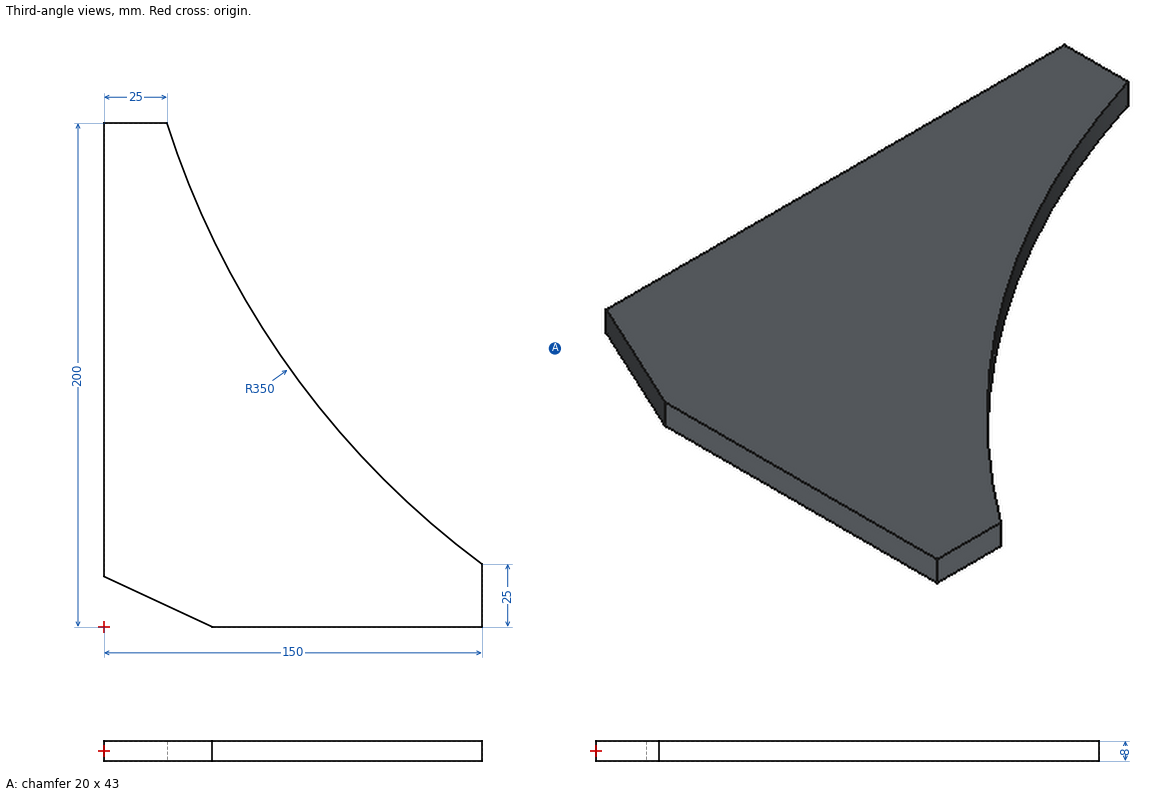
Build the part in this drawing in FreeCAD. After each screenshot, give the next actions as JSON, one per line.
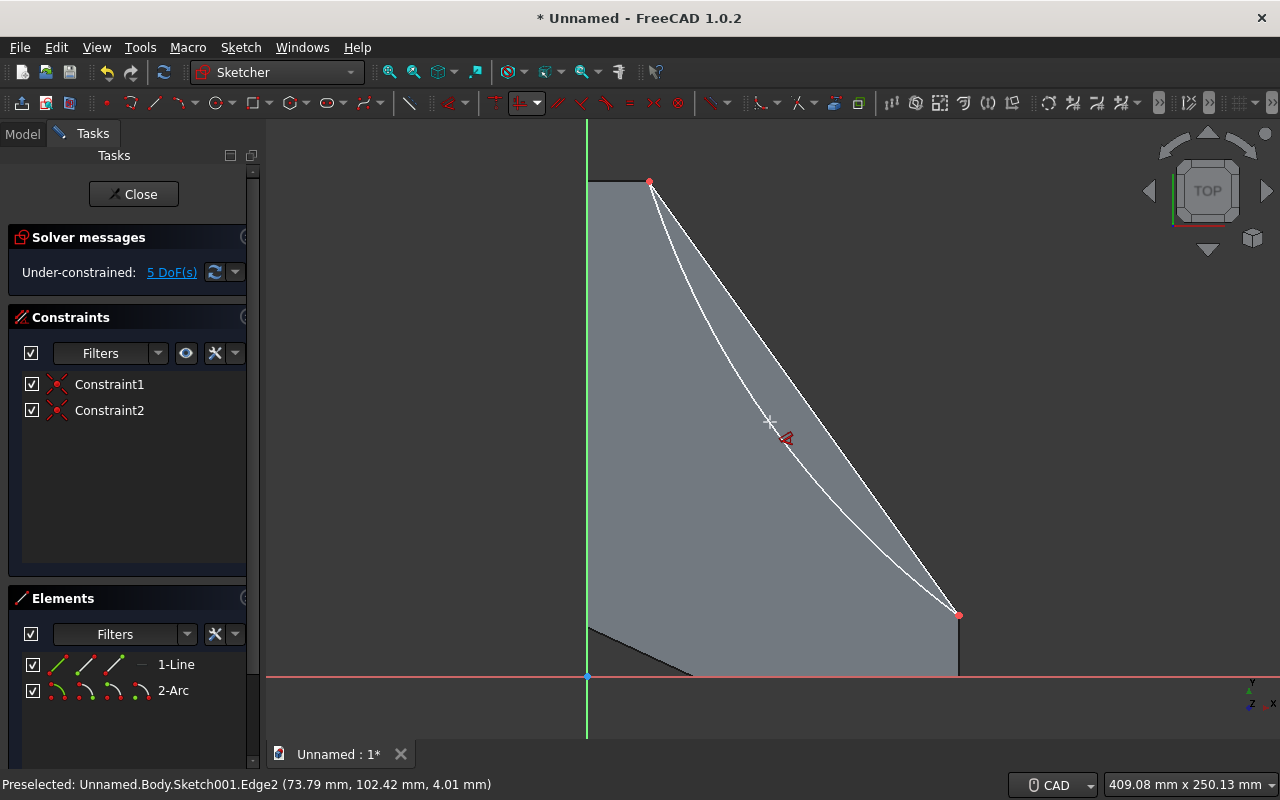
{"action": "left_click", "coordinate": [713, 331]}
{"action": "left_click", "coordinate": [685, 346]}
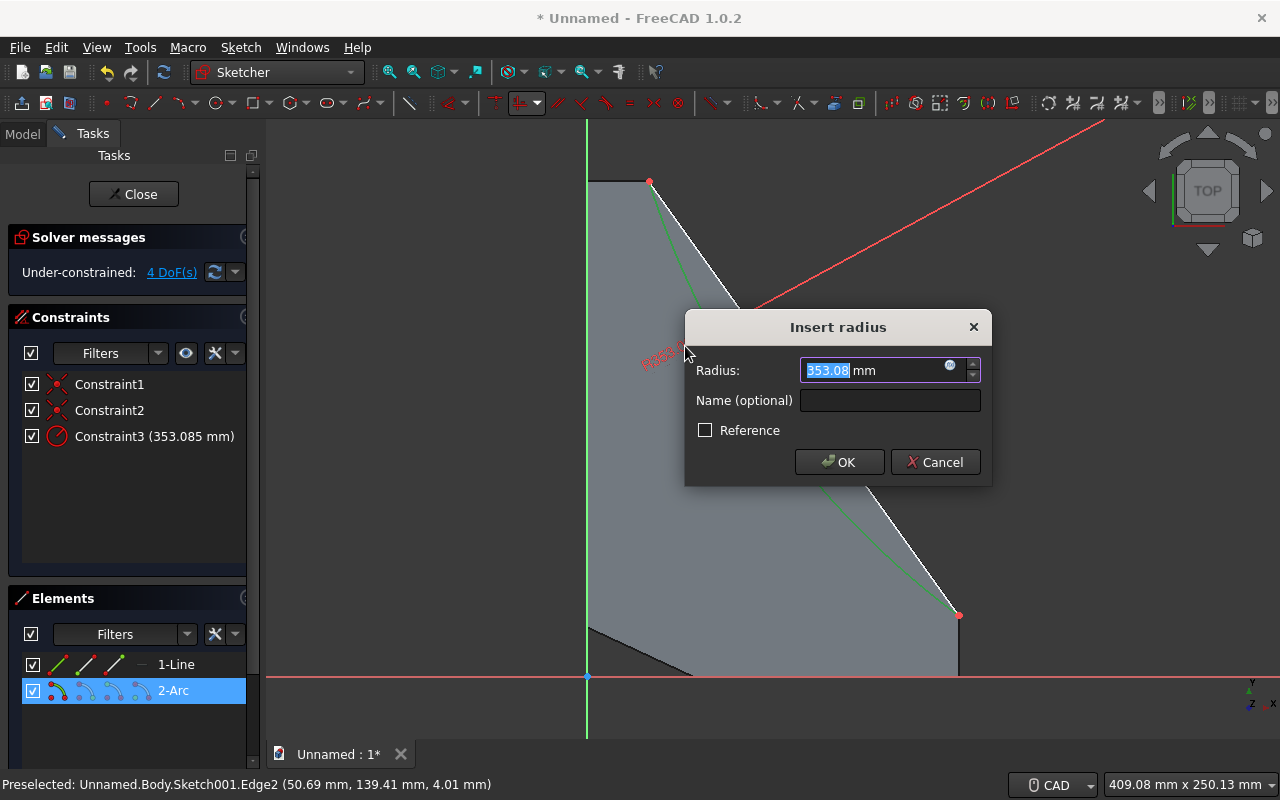
{"action": "type", "text": "350"}
{"action": "key", "text": "Return"}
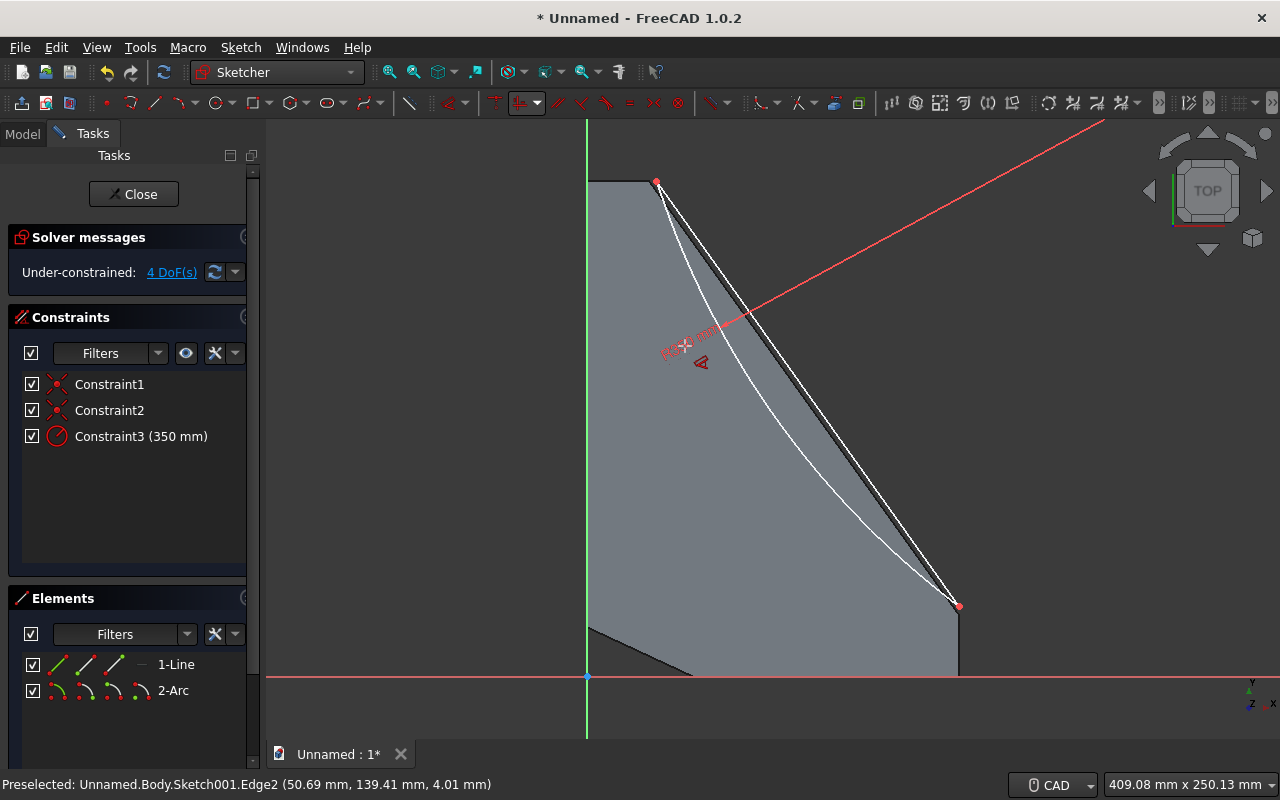
{"action": "left_click", "coordinate": [959, 607]}
{"action": "left_click", "coordinate": [993, 642]}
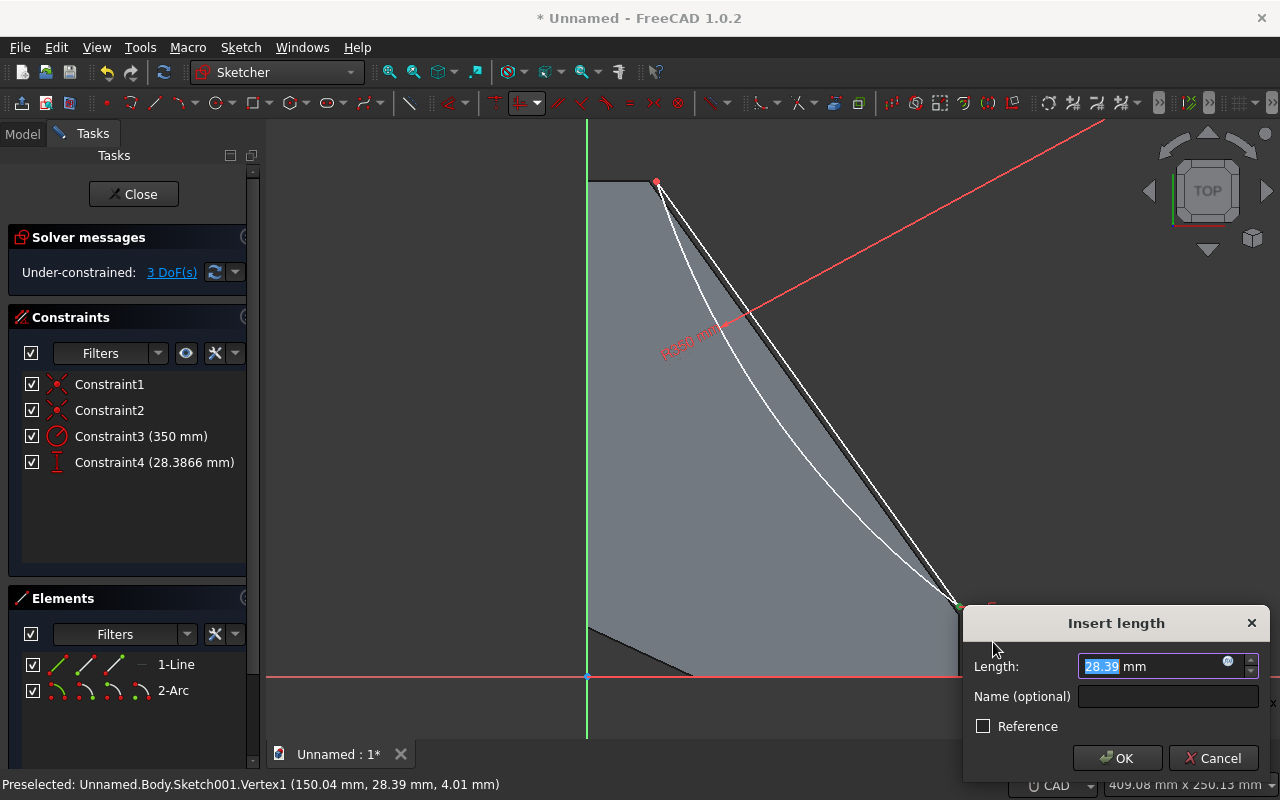
{"action": "type", "text": "25"}
{"action": "key", "text": "Return"}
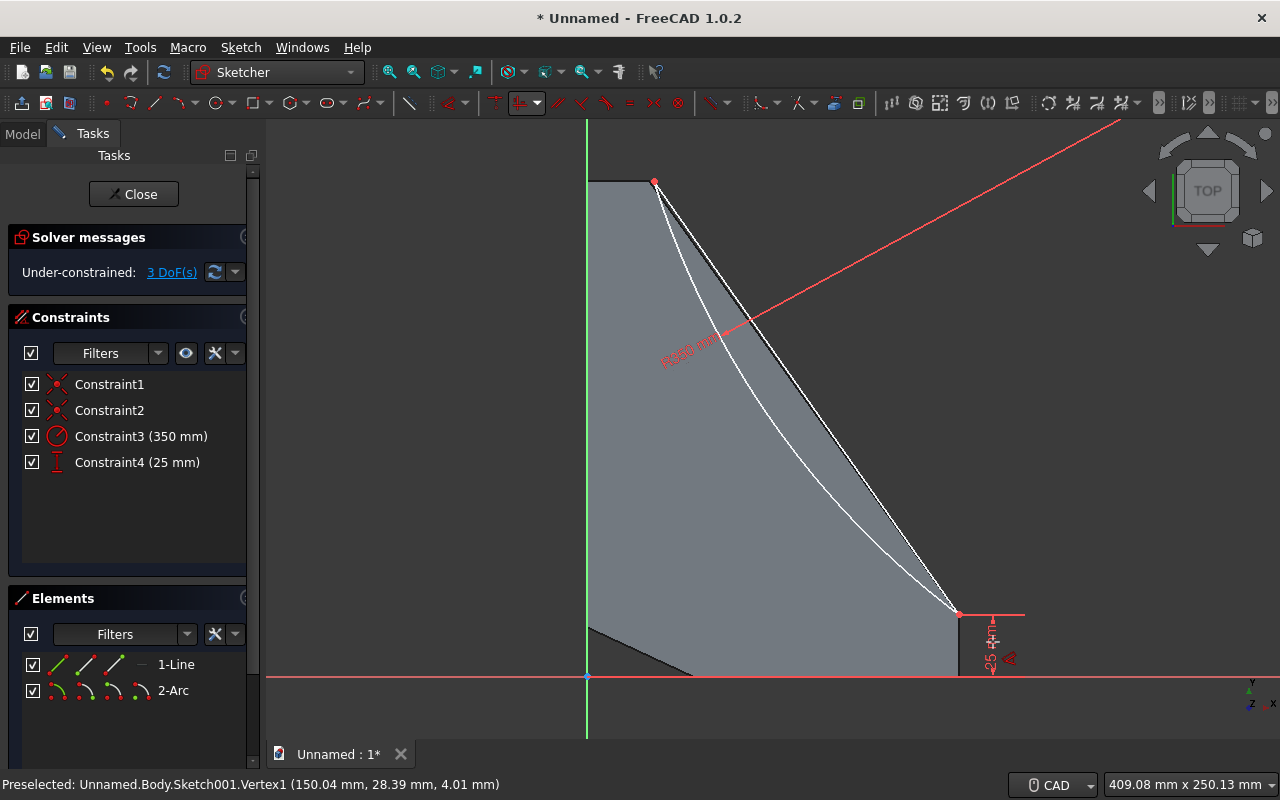
{"action": "left_click", "coordinate": [654, 182]}
{"action": "left_click", "coordinate": [621, 711]}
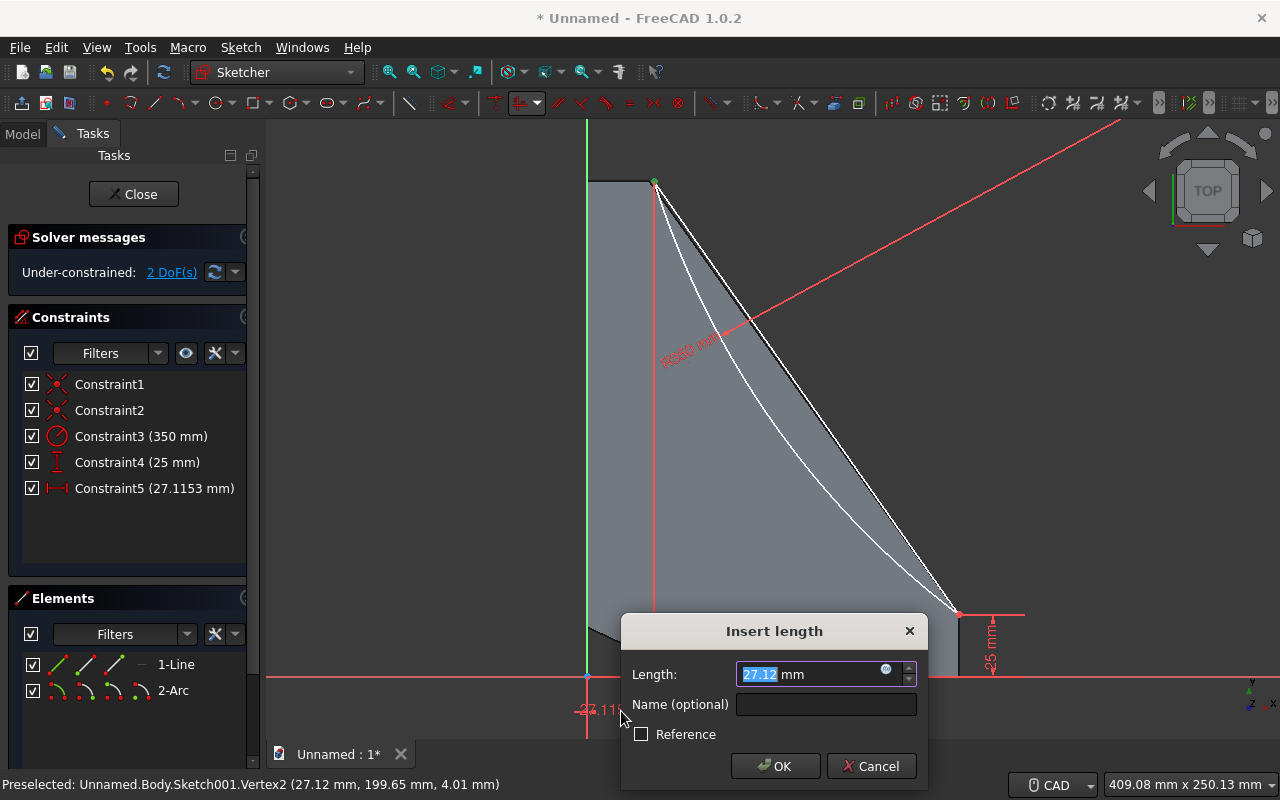
{"action": "type", "text": "25"}
{"action": "key", "text": "Return"}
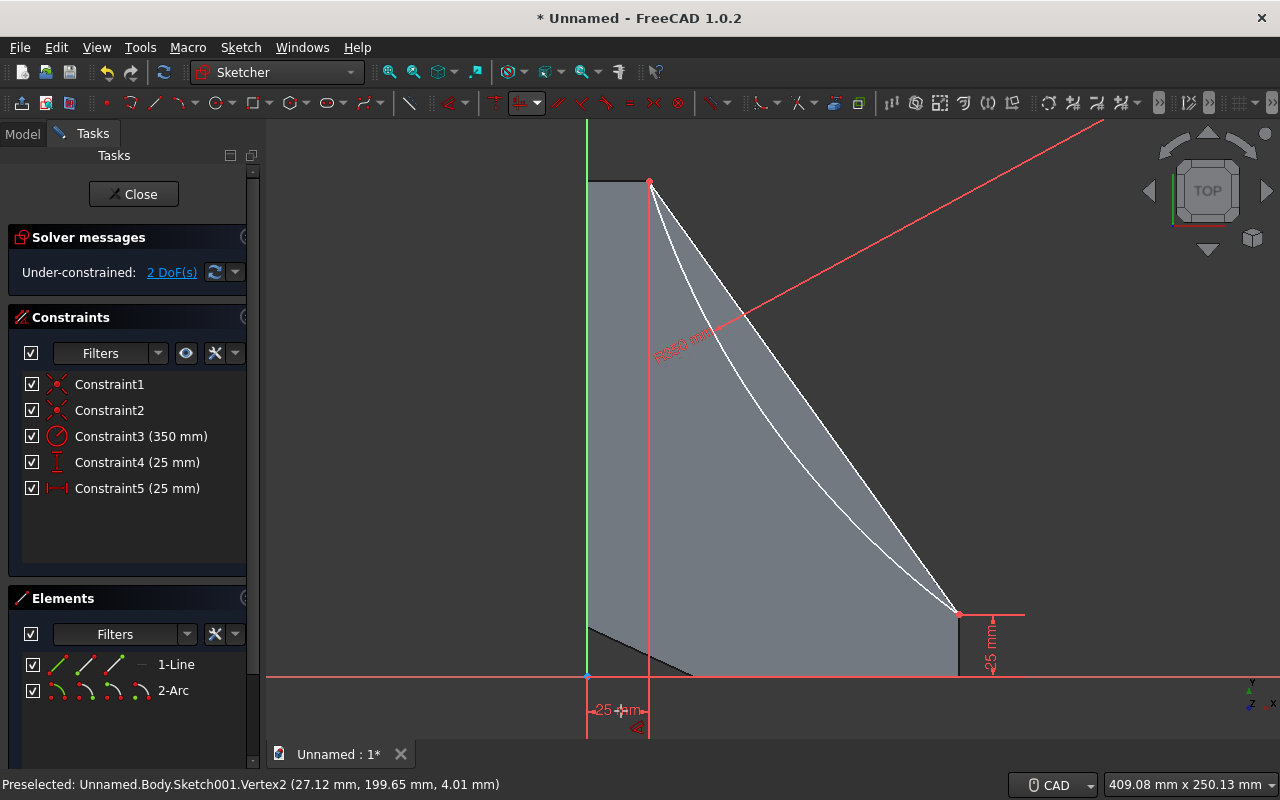
{"action": "left_click", "coordinate": [959, 615]}
{"action": "left_click", "coordinate": [773, 711]}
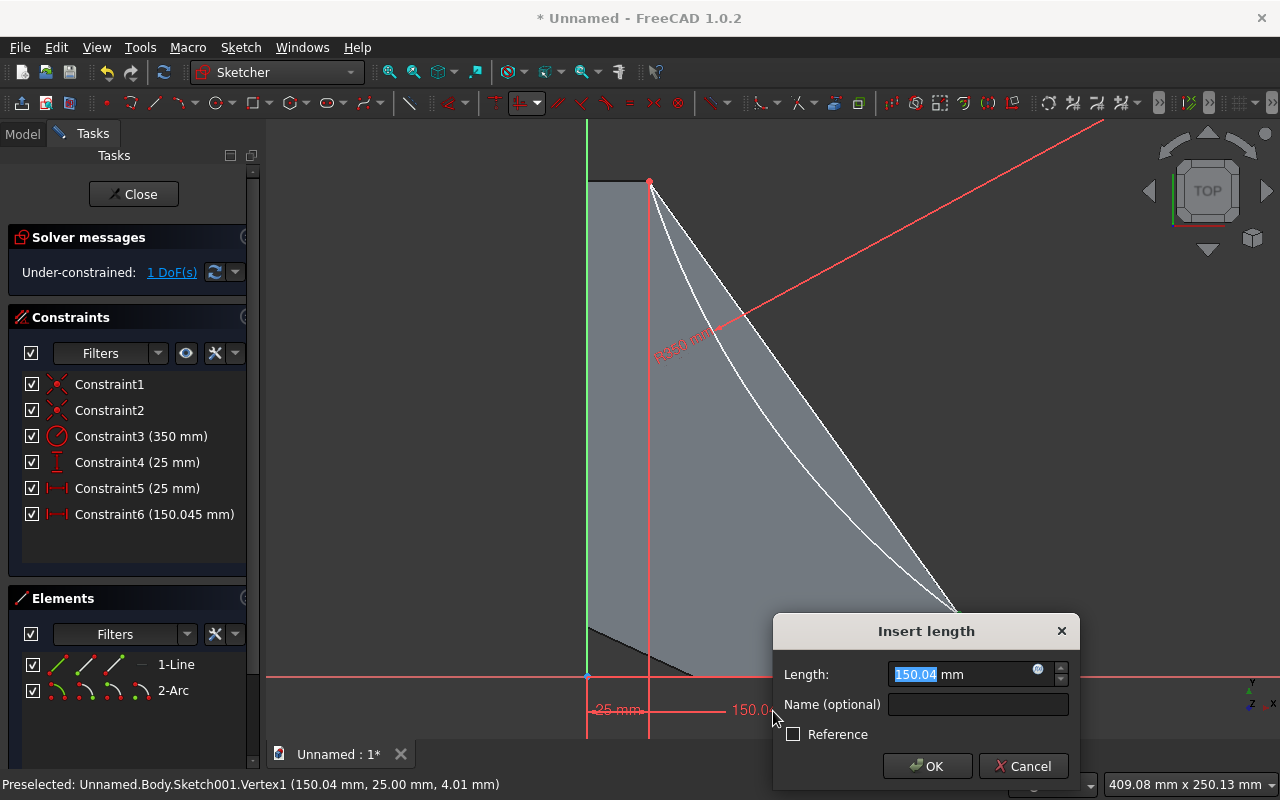
{"action": "type", "text": "150"}
{"action": "key", "text": "Return"}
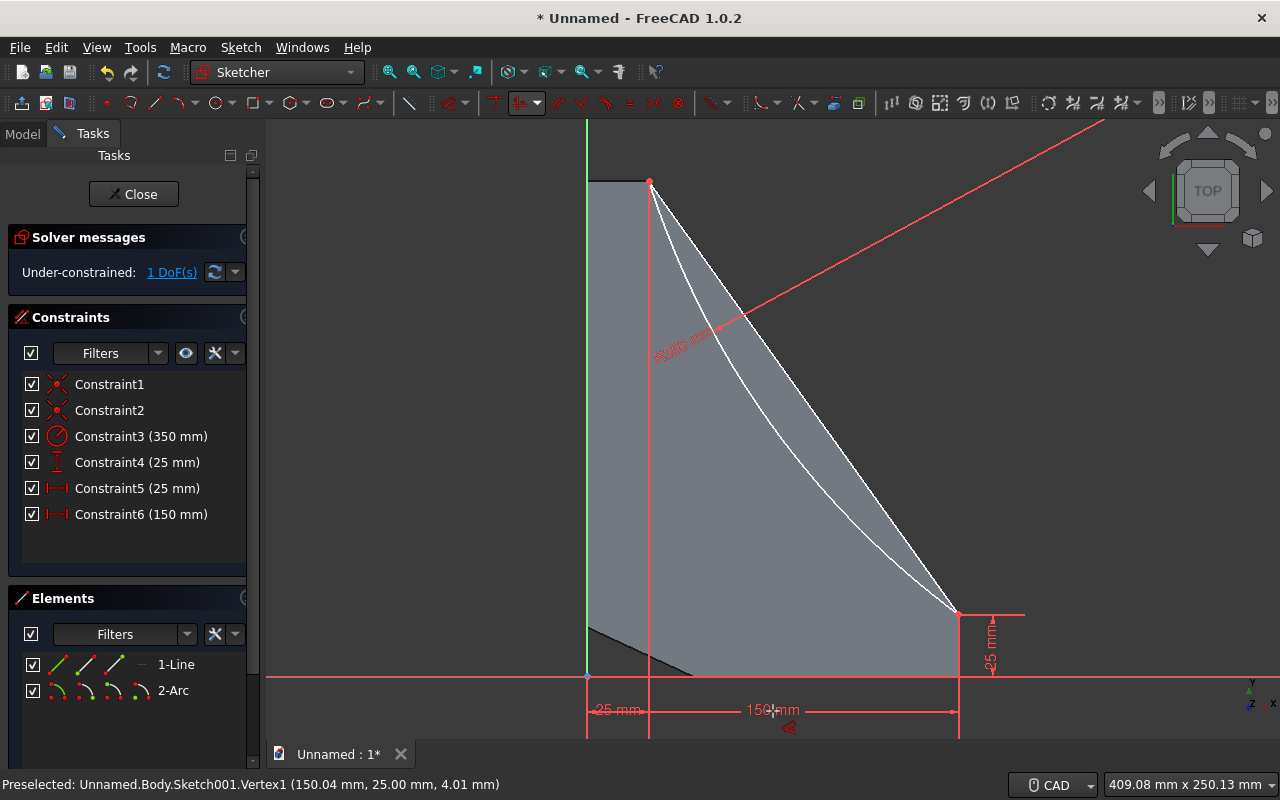
{"action": "left_click", "coordinate": [649, 182]}
{"action": "left_click", "coordinate": [553, 429]}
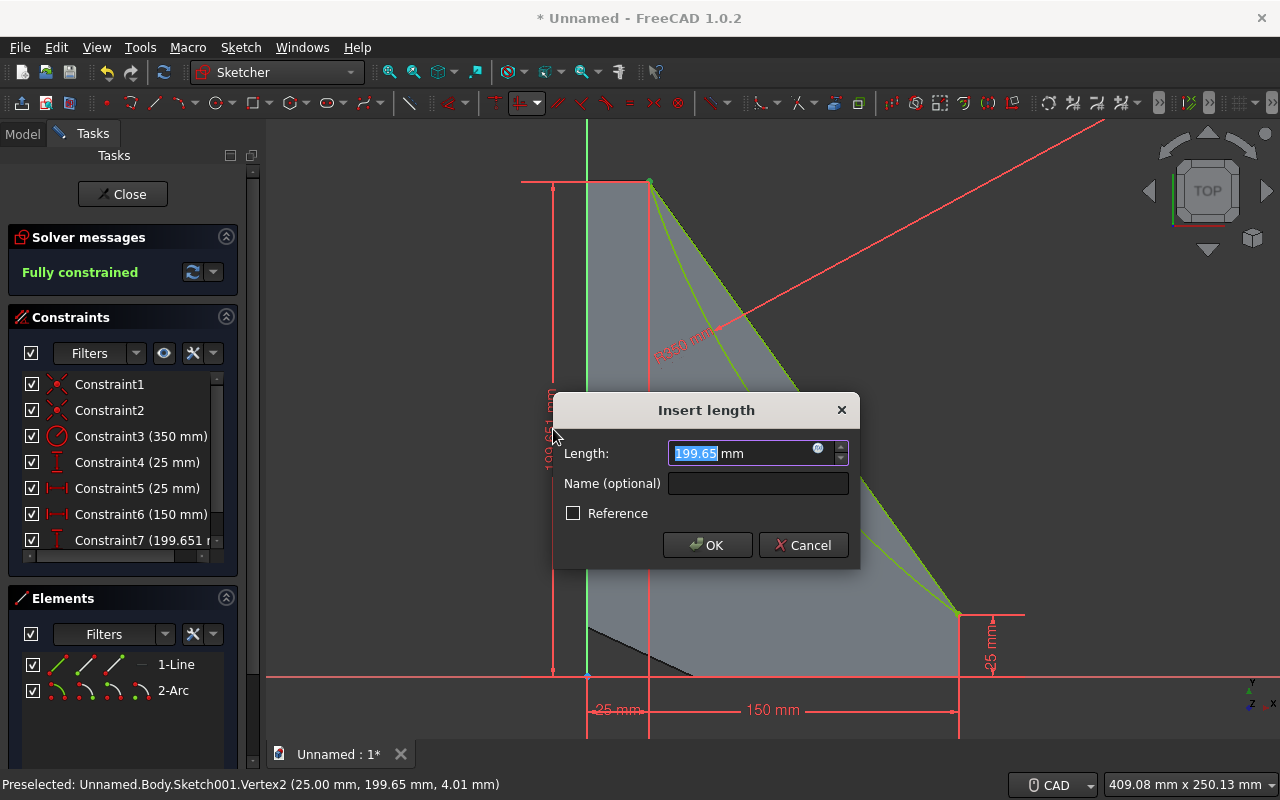
{"action": "type", "text": "200"}
{"action": "key", "text": "Return"}
{"action": "key", "text": "Escape"}